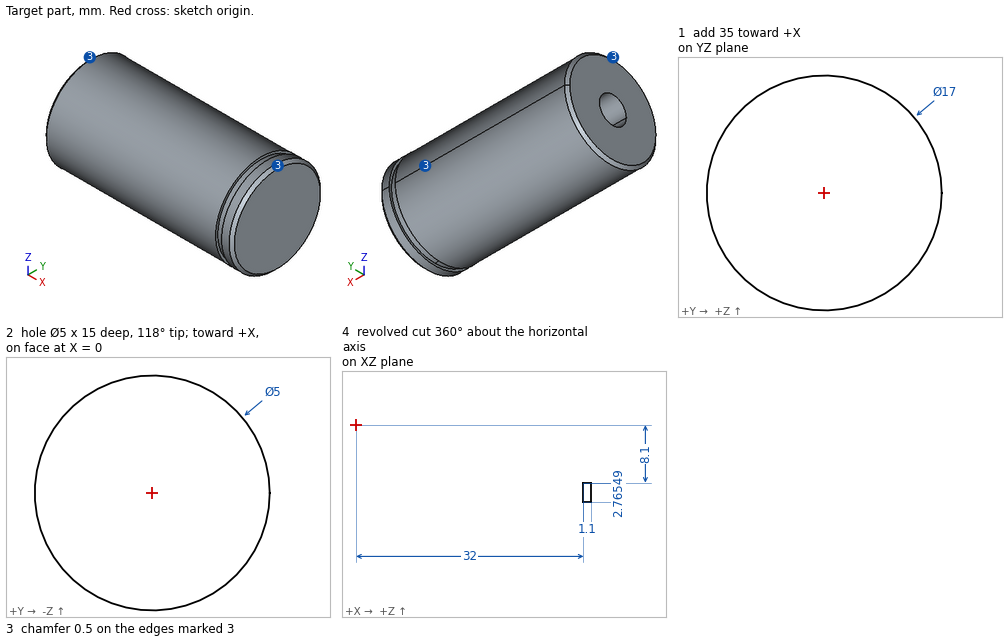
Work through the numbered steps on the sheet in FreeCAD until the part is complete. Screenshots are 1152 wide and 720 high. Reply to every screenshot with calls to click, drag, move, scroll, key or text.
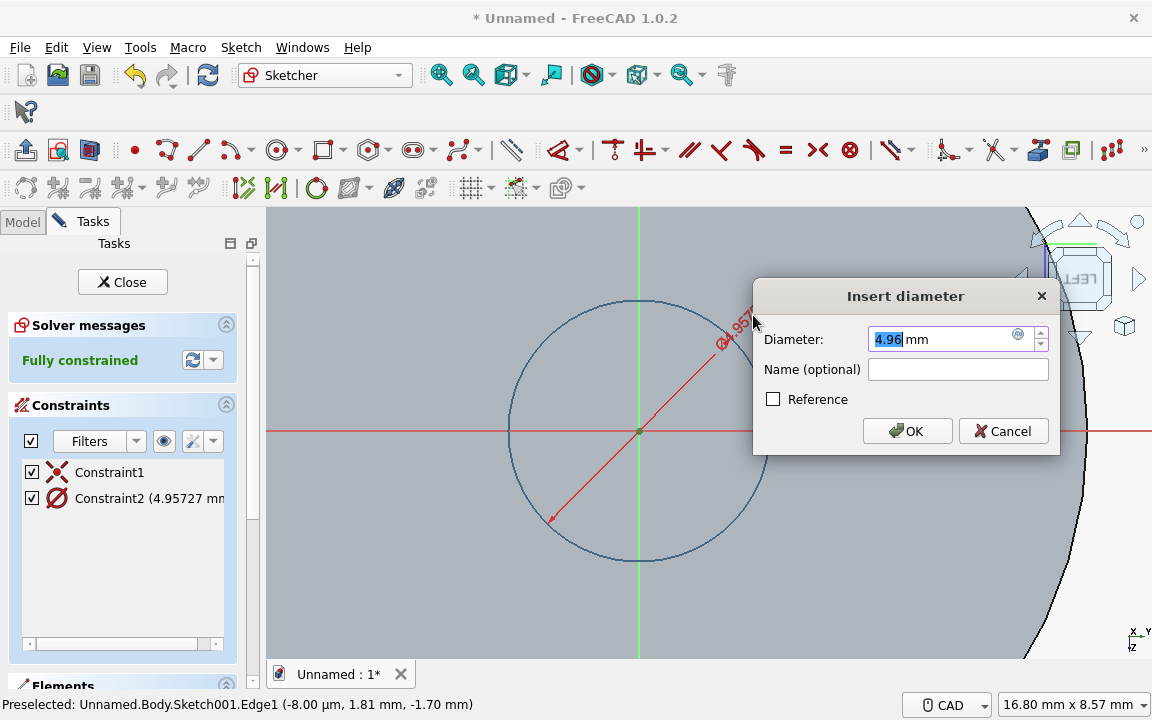
text(5)
key(Return)
key(Escape)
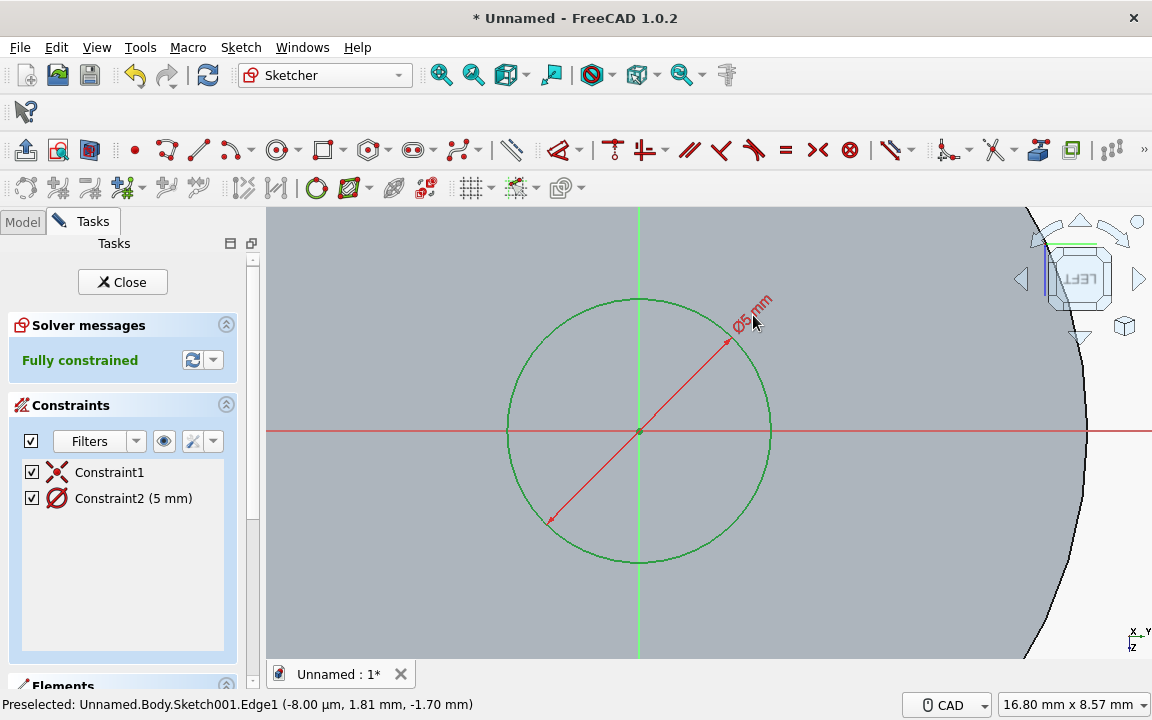
click(123, 282)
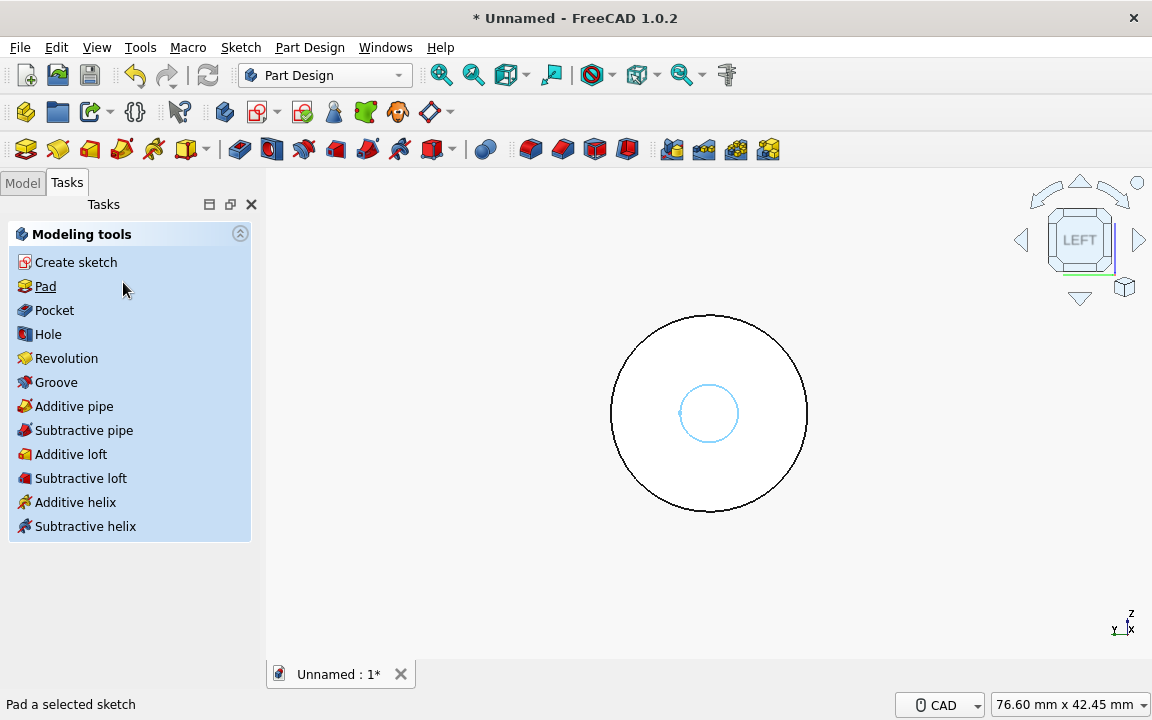
click(272, 150)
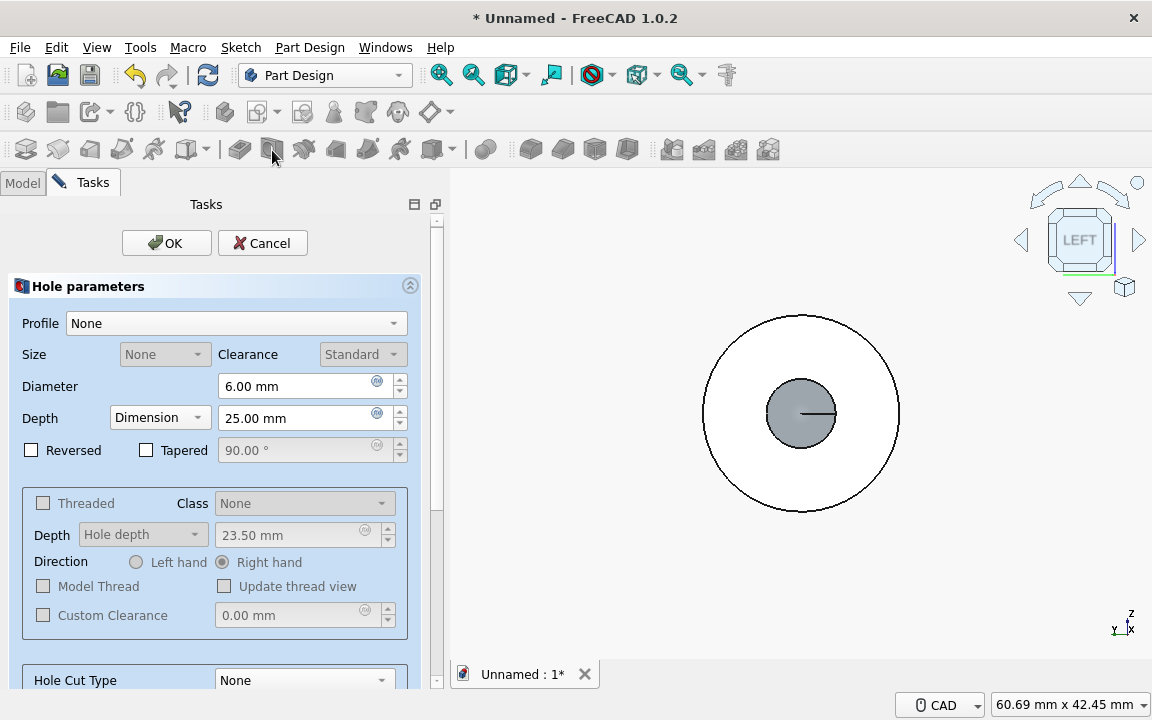
triple_click(305, 386)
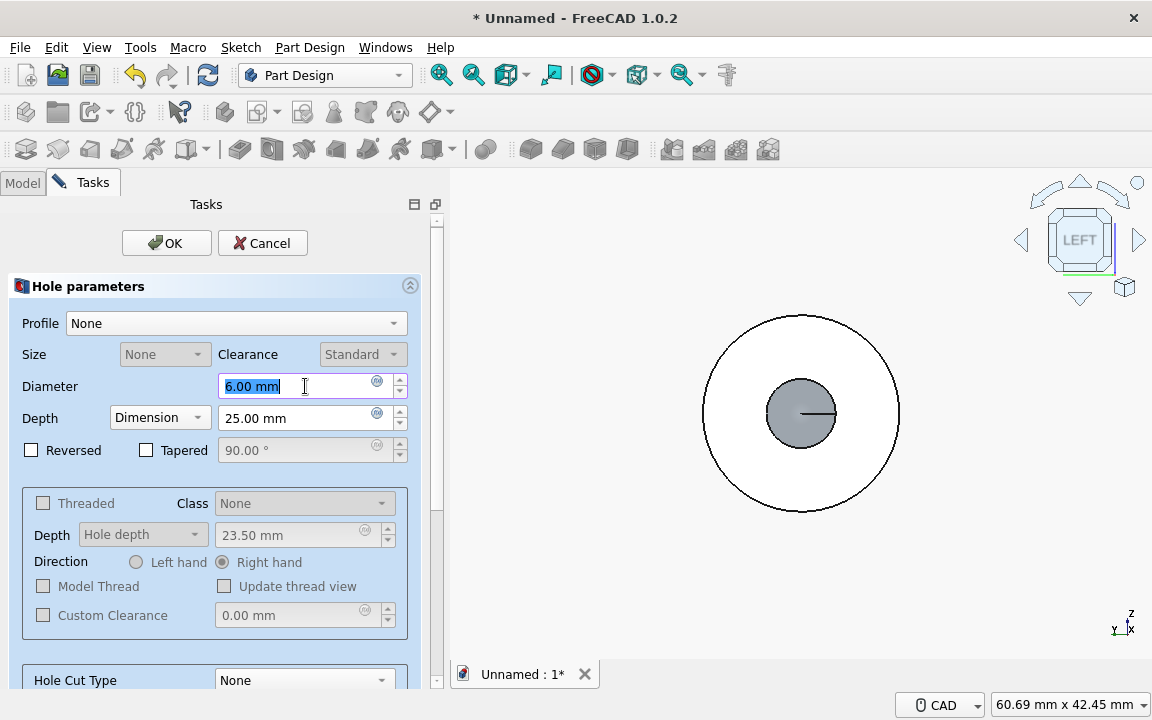
text(5)
key(Tab)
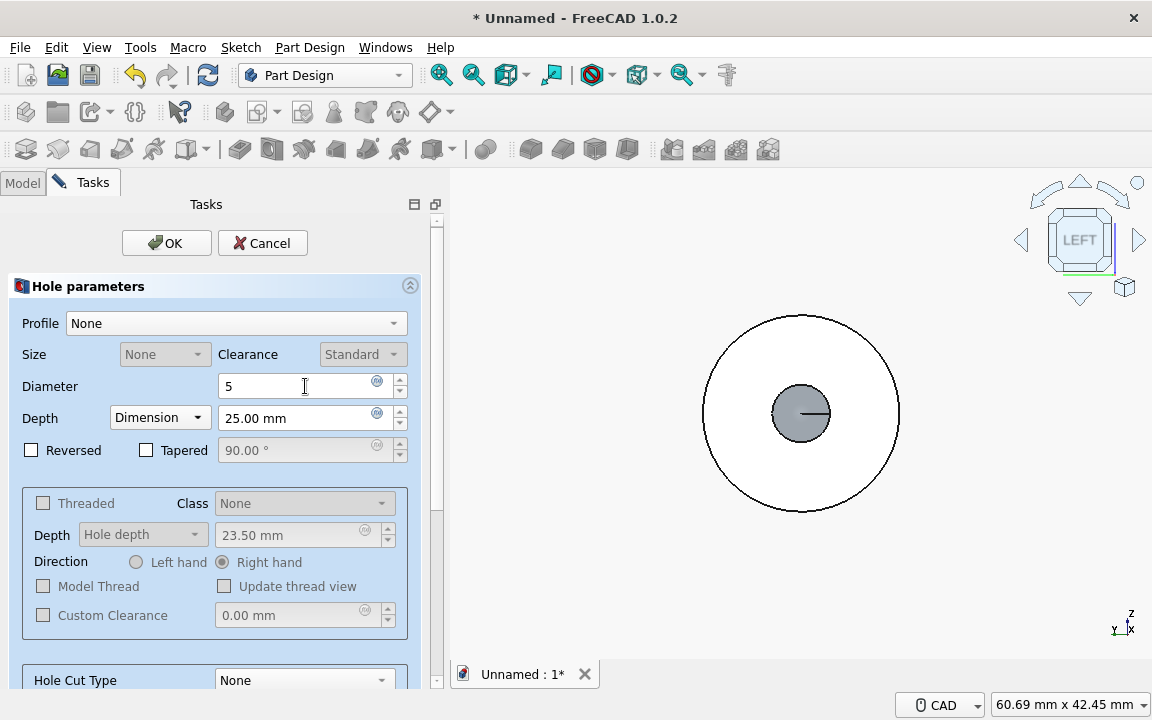
triple_click(305, 418)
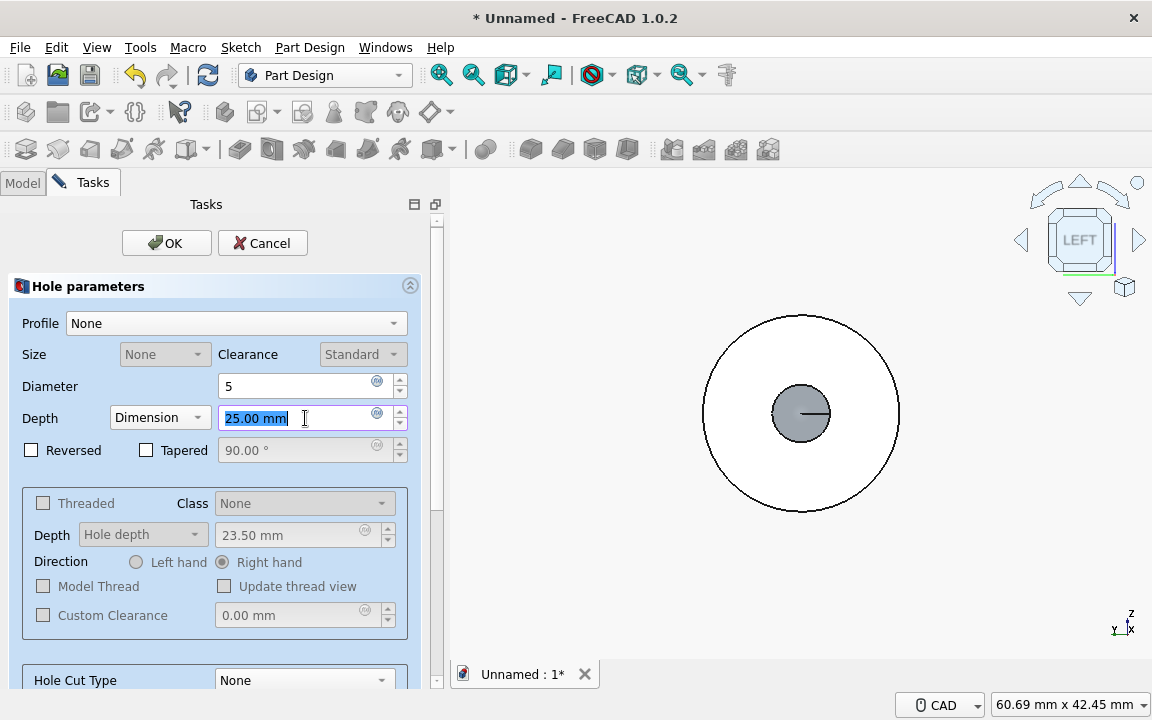
text(15)
key(Tab)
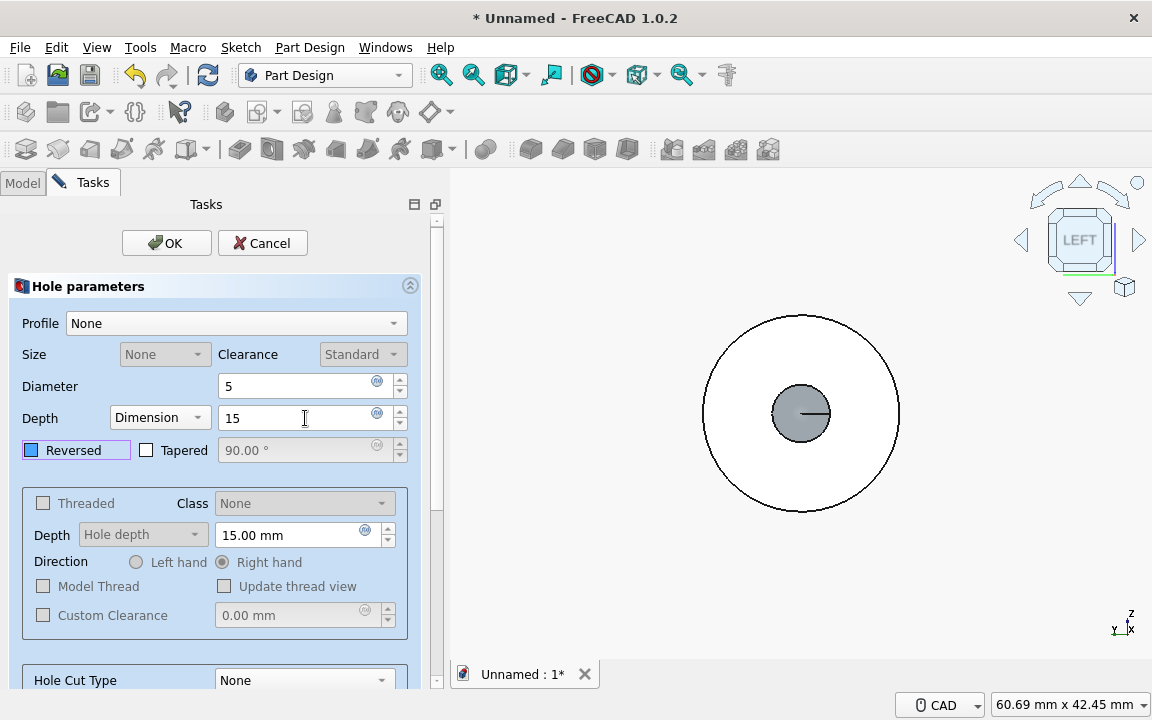
click(167, 243)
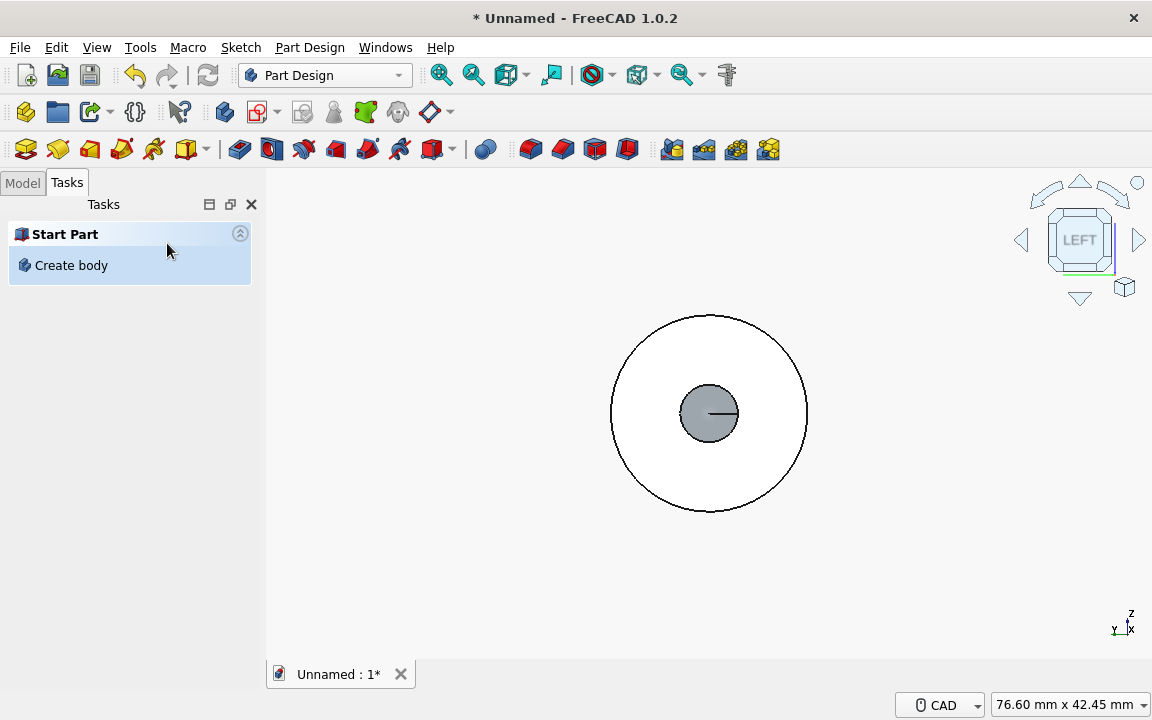
click(442, 76)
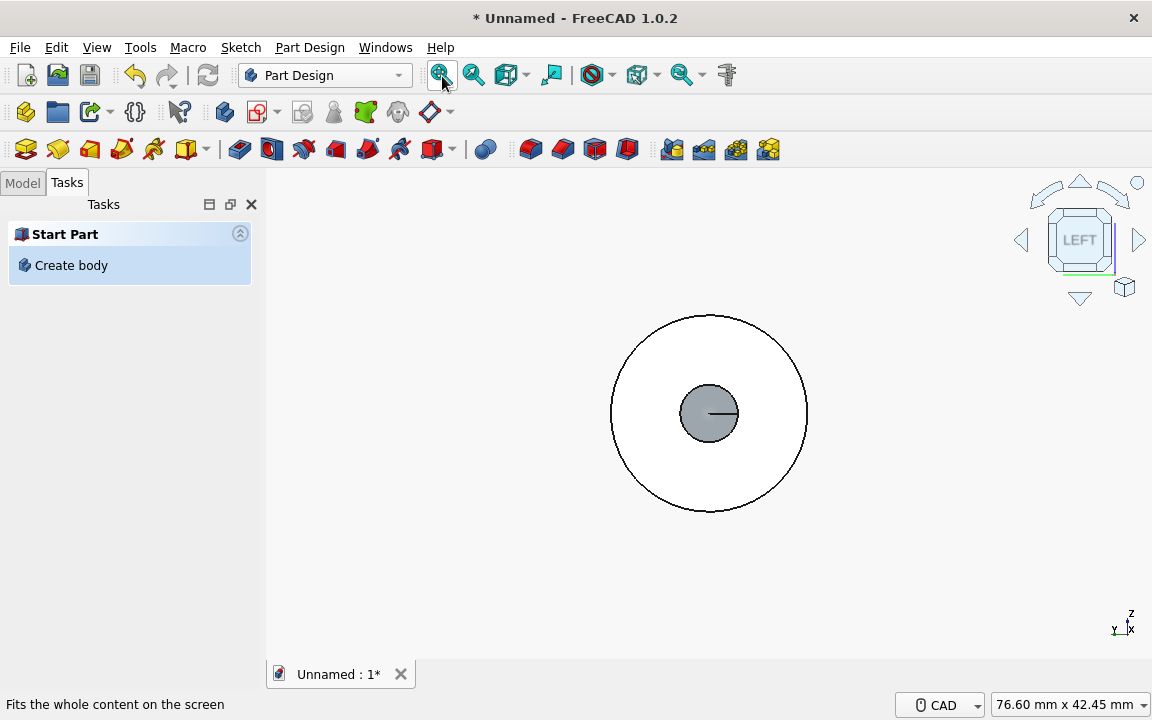
click(789, 355)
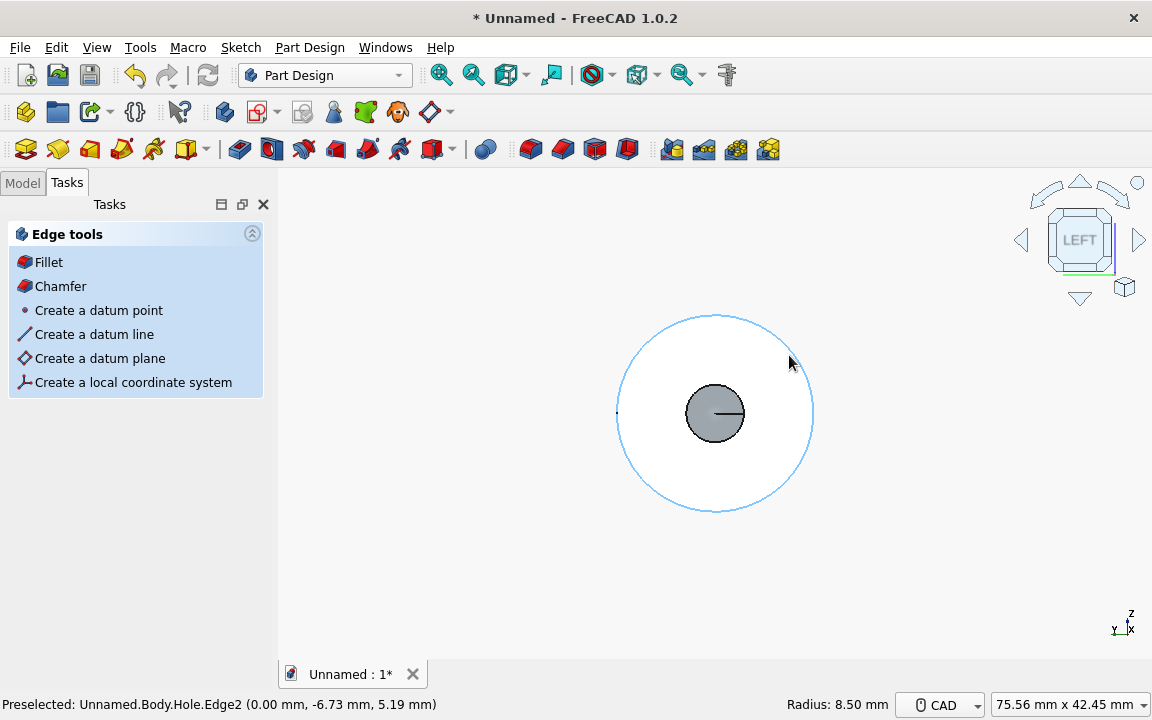
key(0)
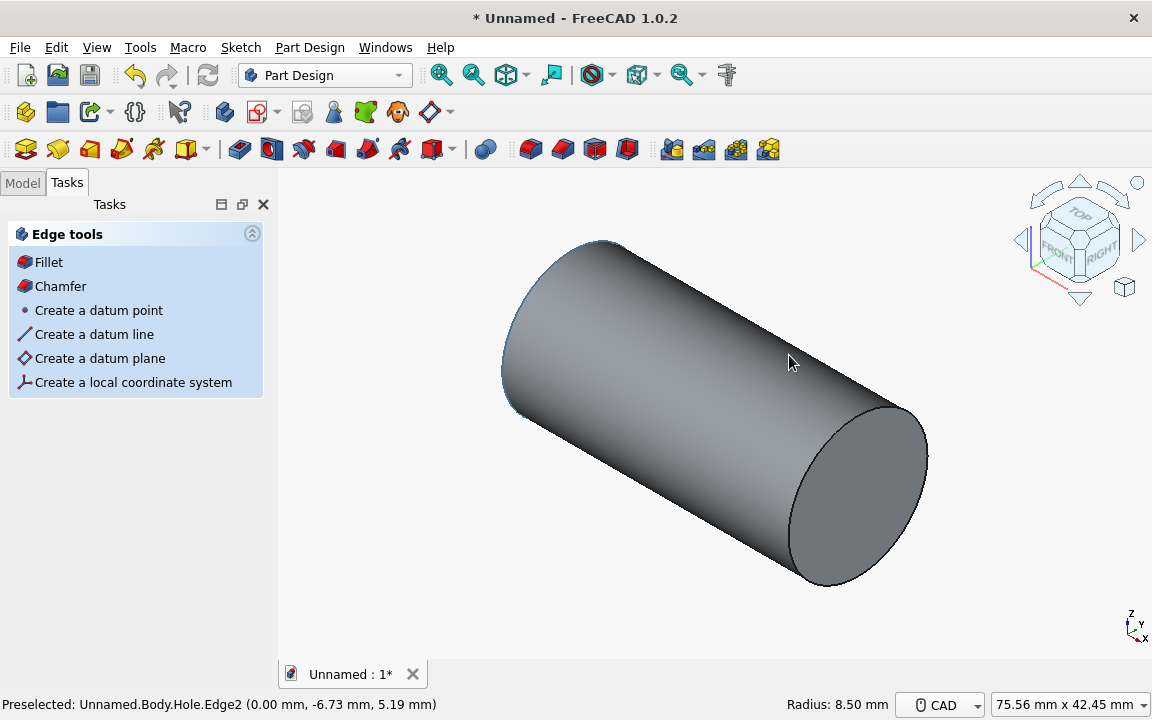
click(789, 535, ctrl)